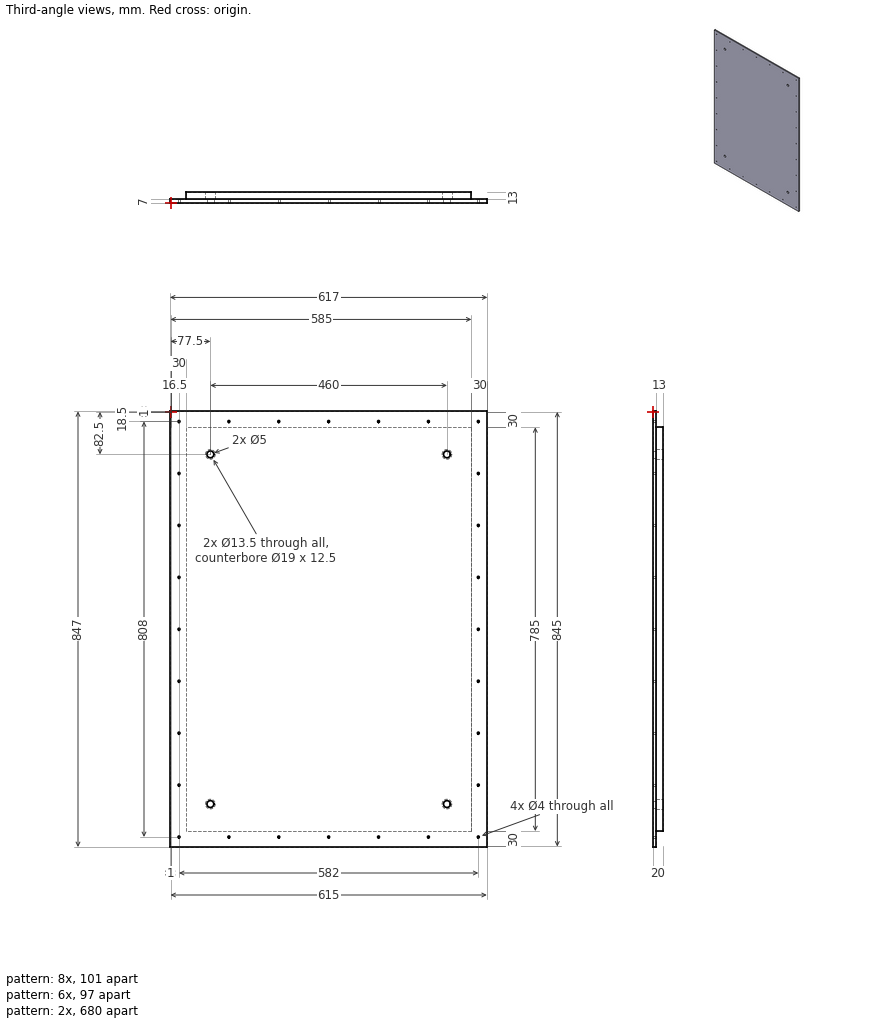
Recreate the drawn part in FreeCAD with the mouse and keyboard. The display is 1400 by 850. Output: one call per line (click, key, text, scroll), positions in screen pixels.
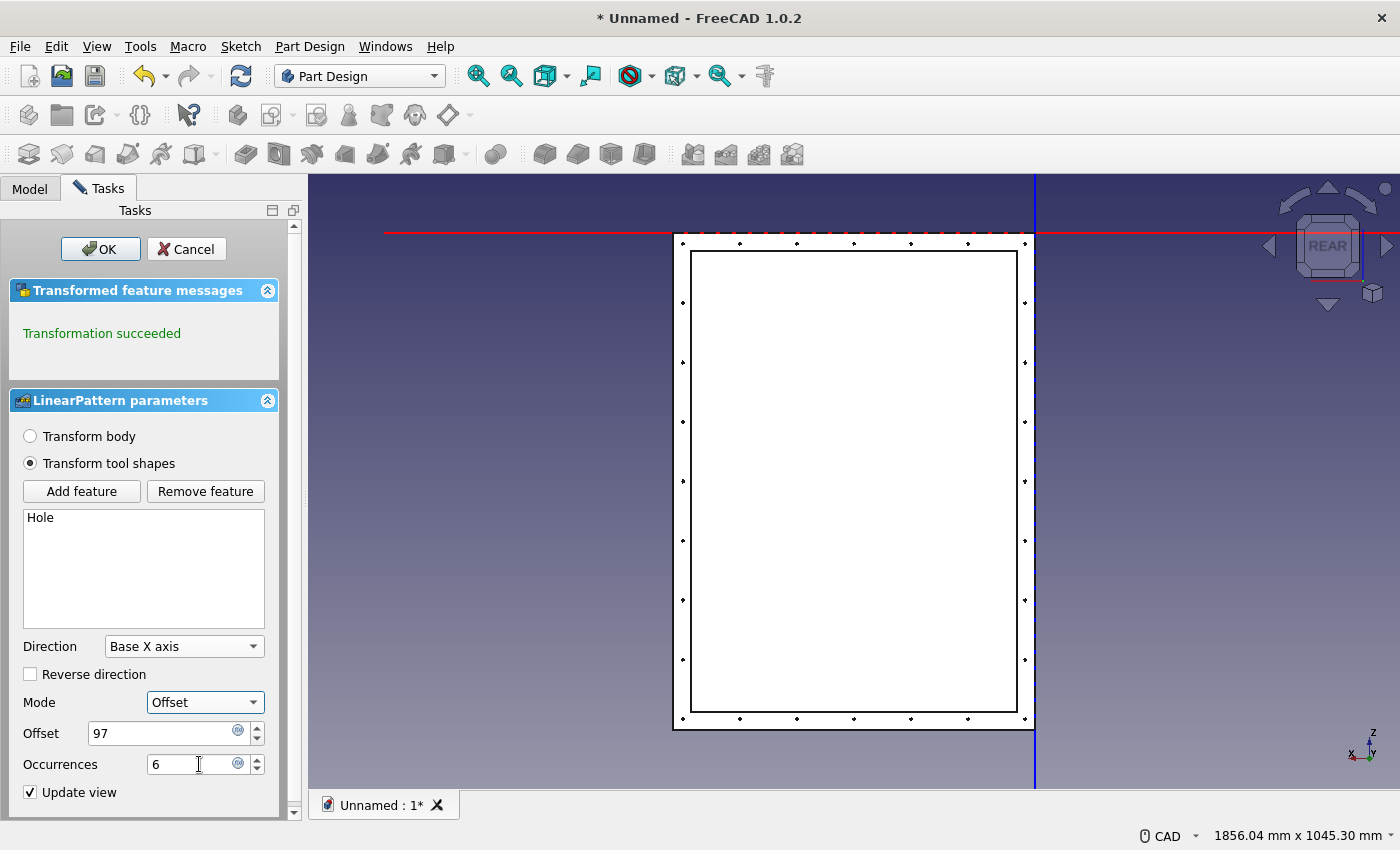
click(101, 249)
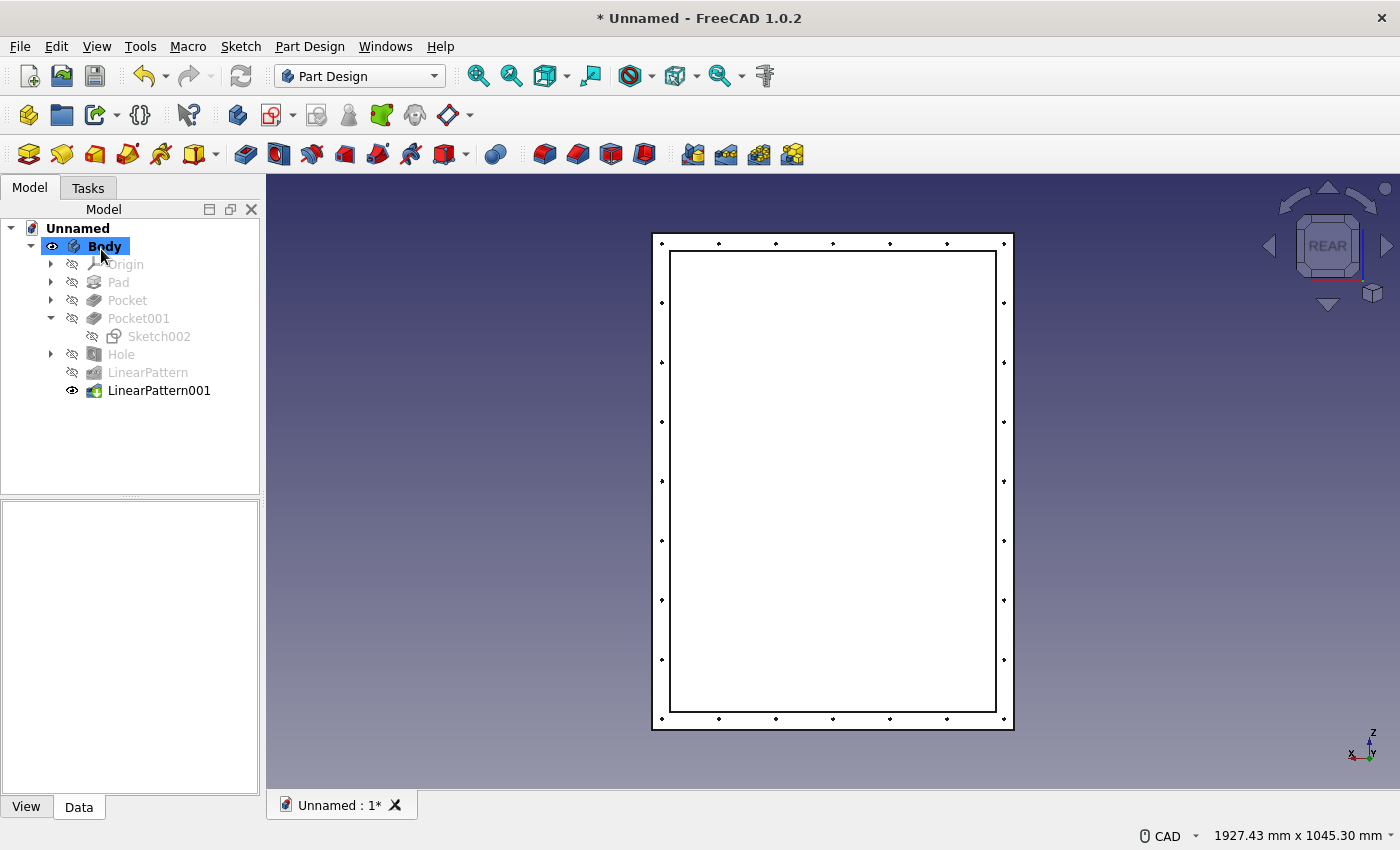
click(661, 500)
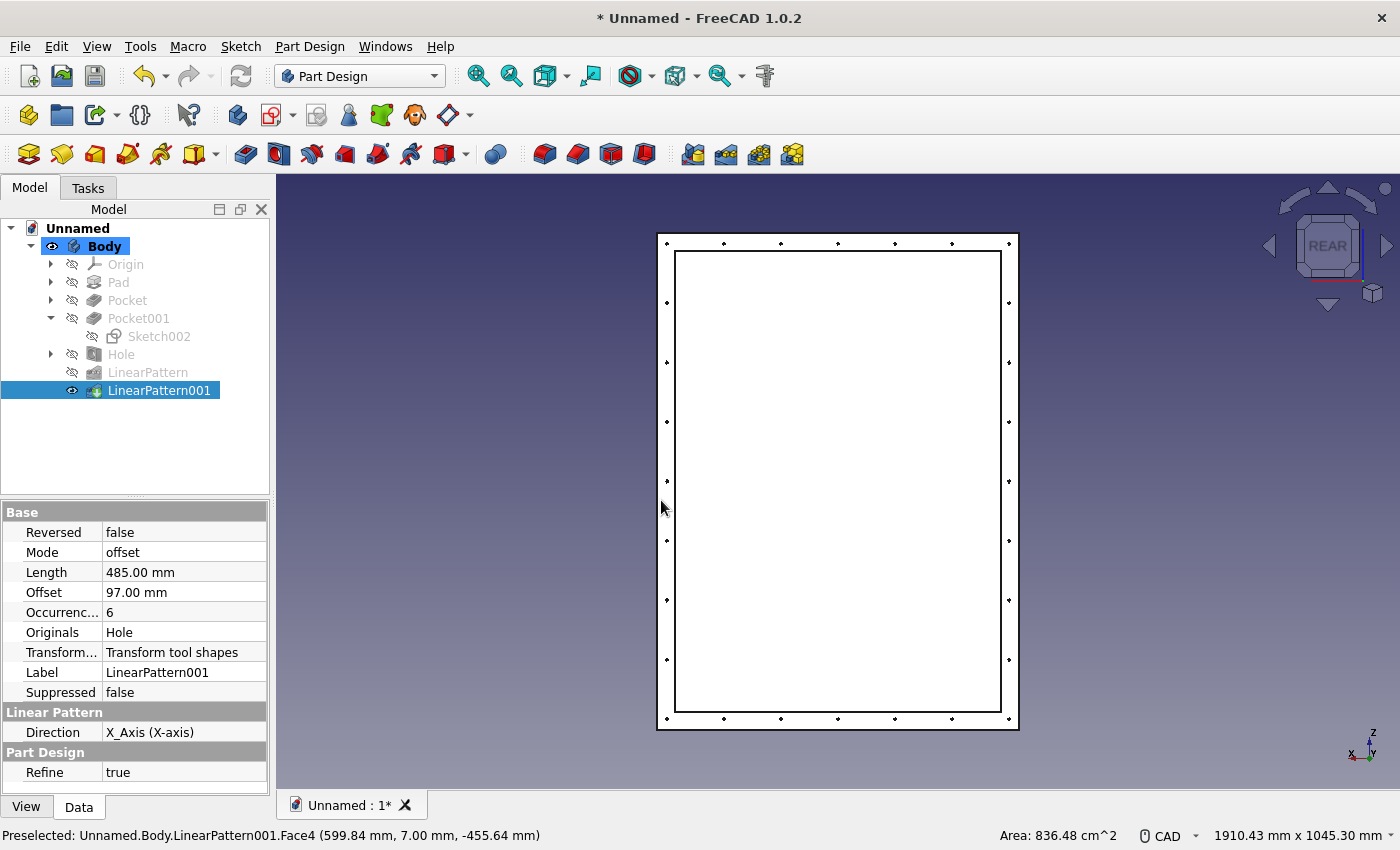
click(270, 116)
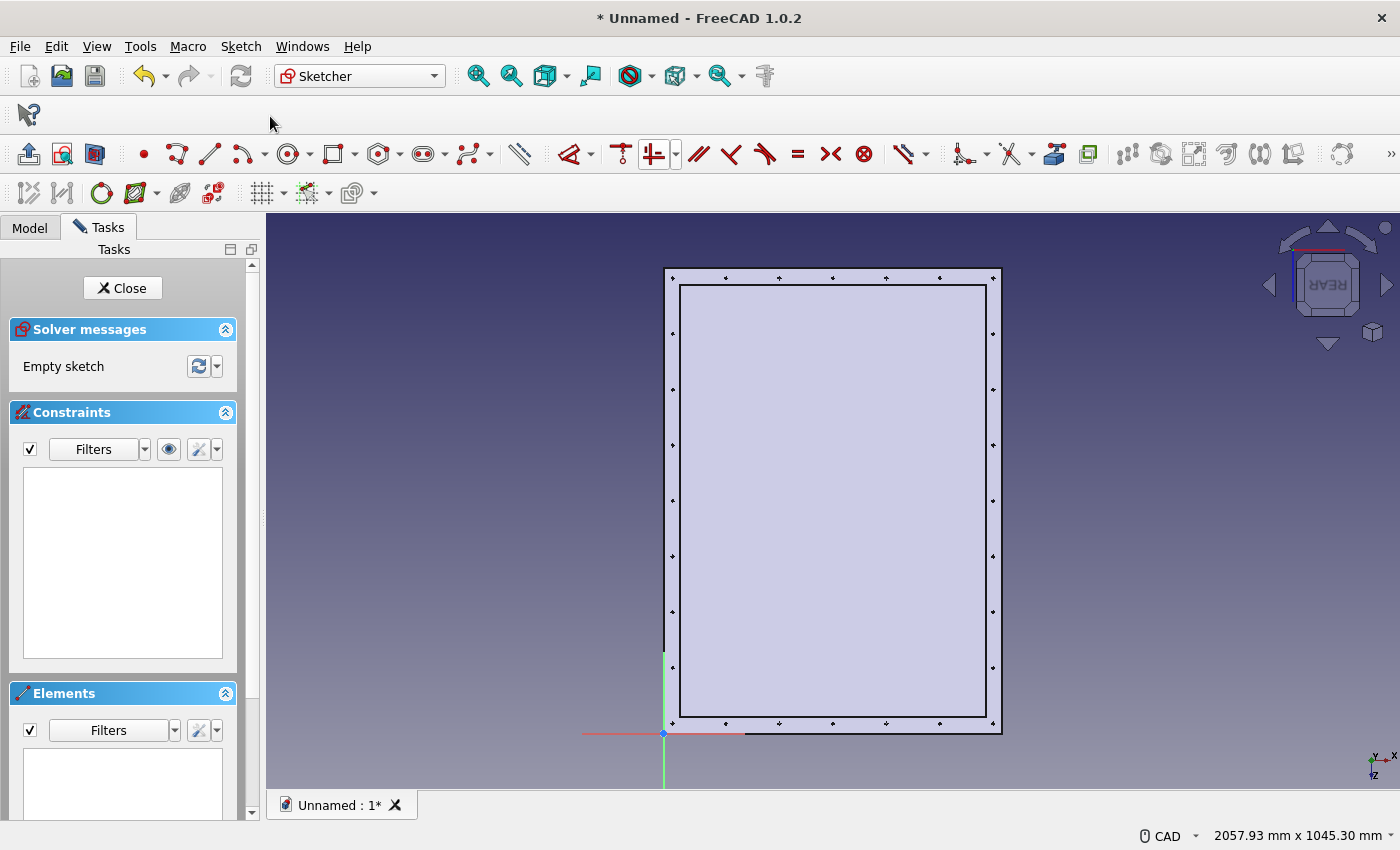
click(332, 154)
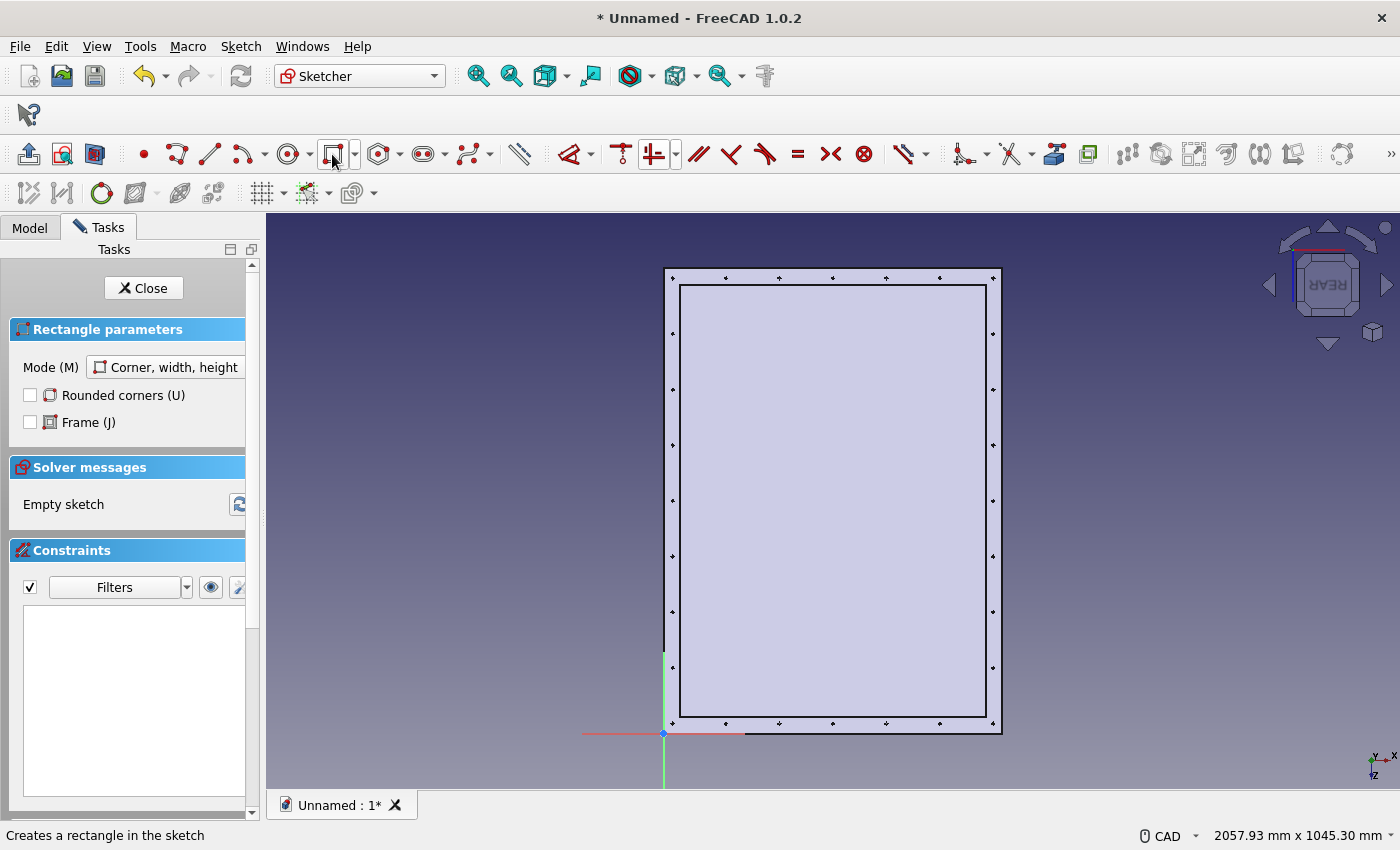
scroll(663, 268, up, 17)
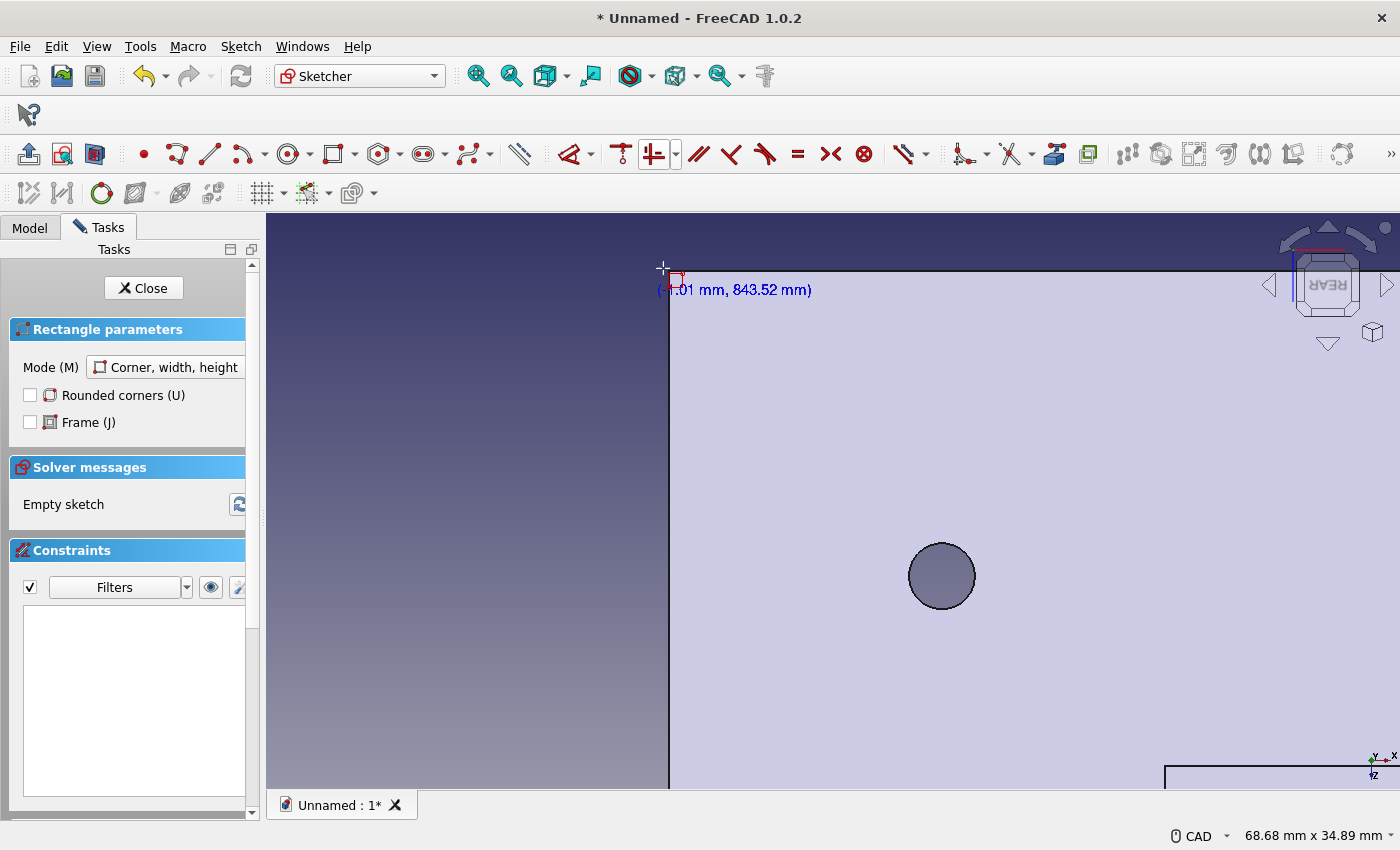
click(653, 254)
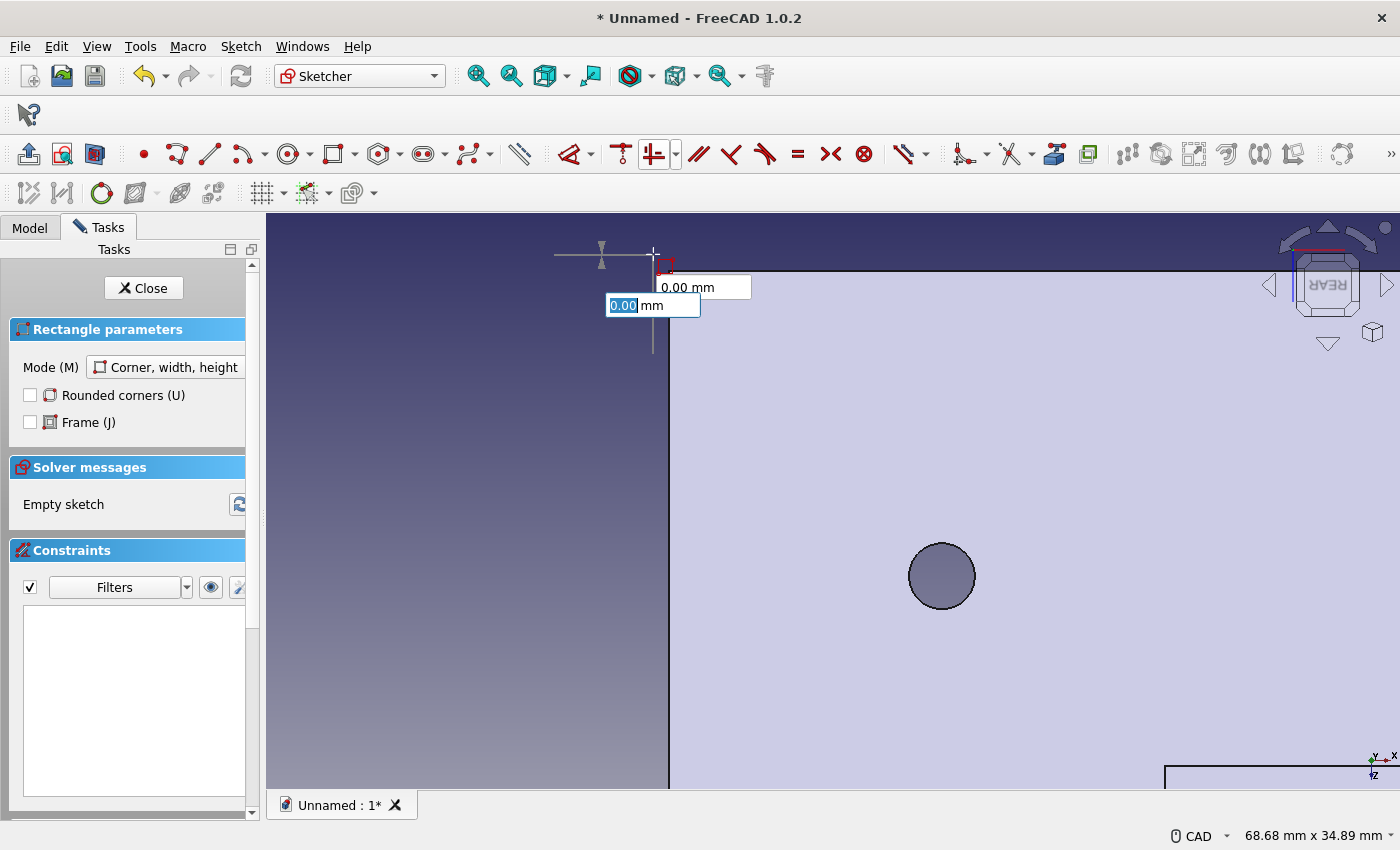
scroll(592, 268, down, 17)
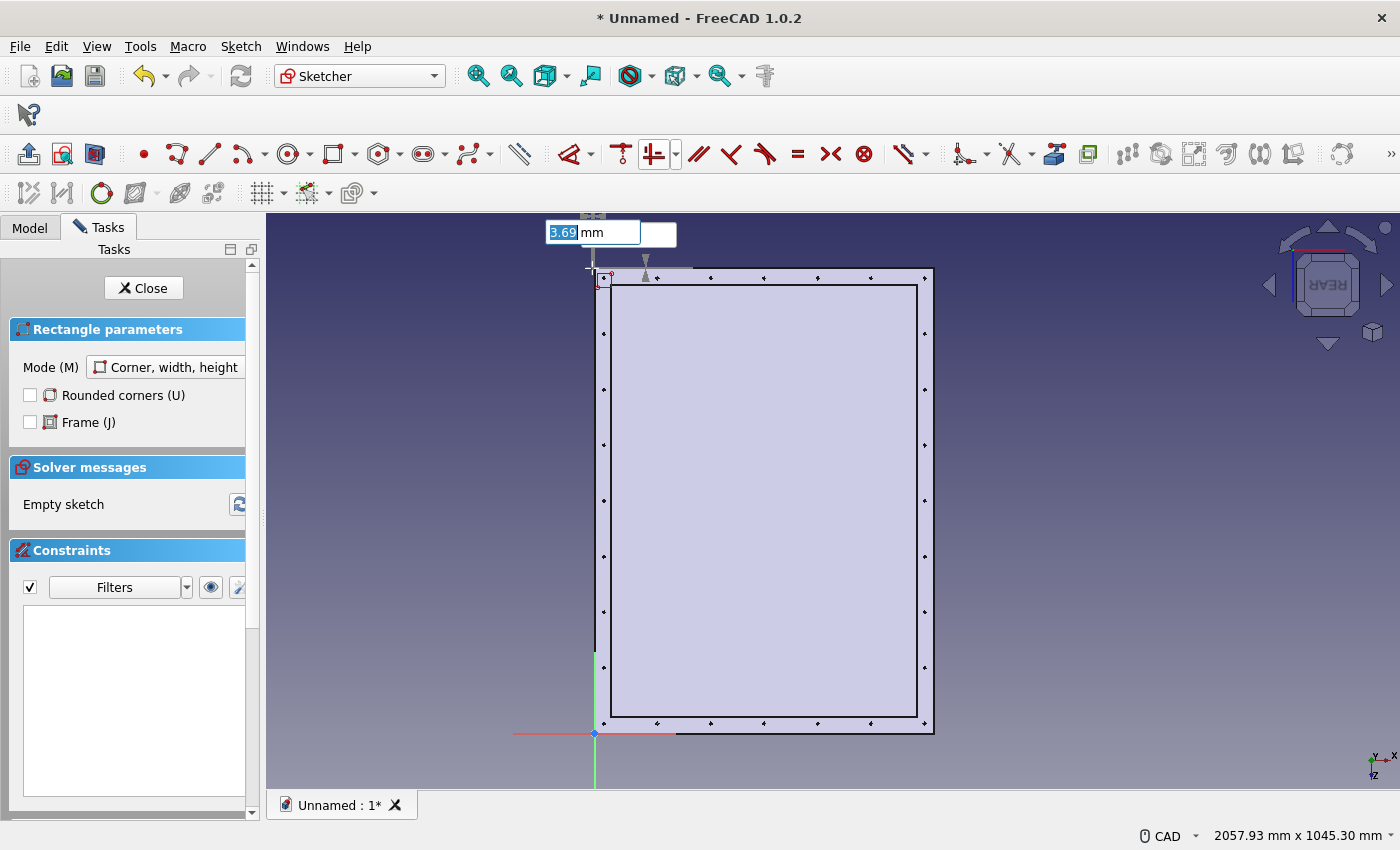
scroll(934, 734, up, 17)